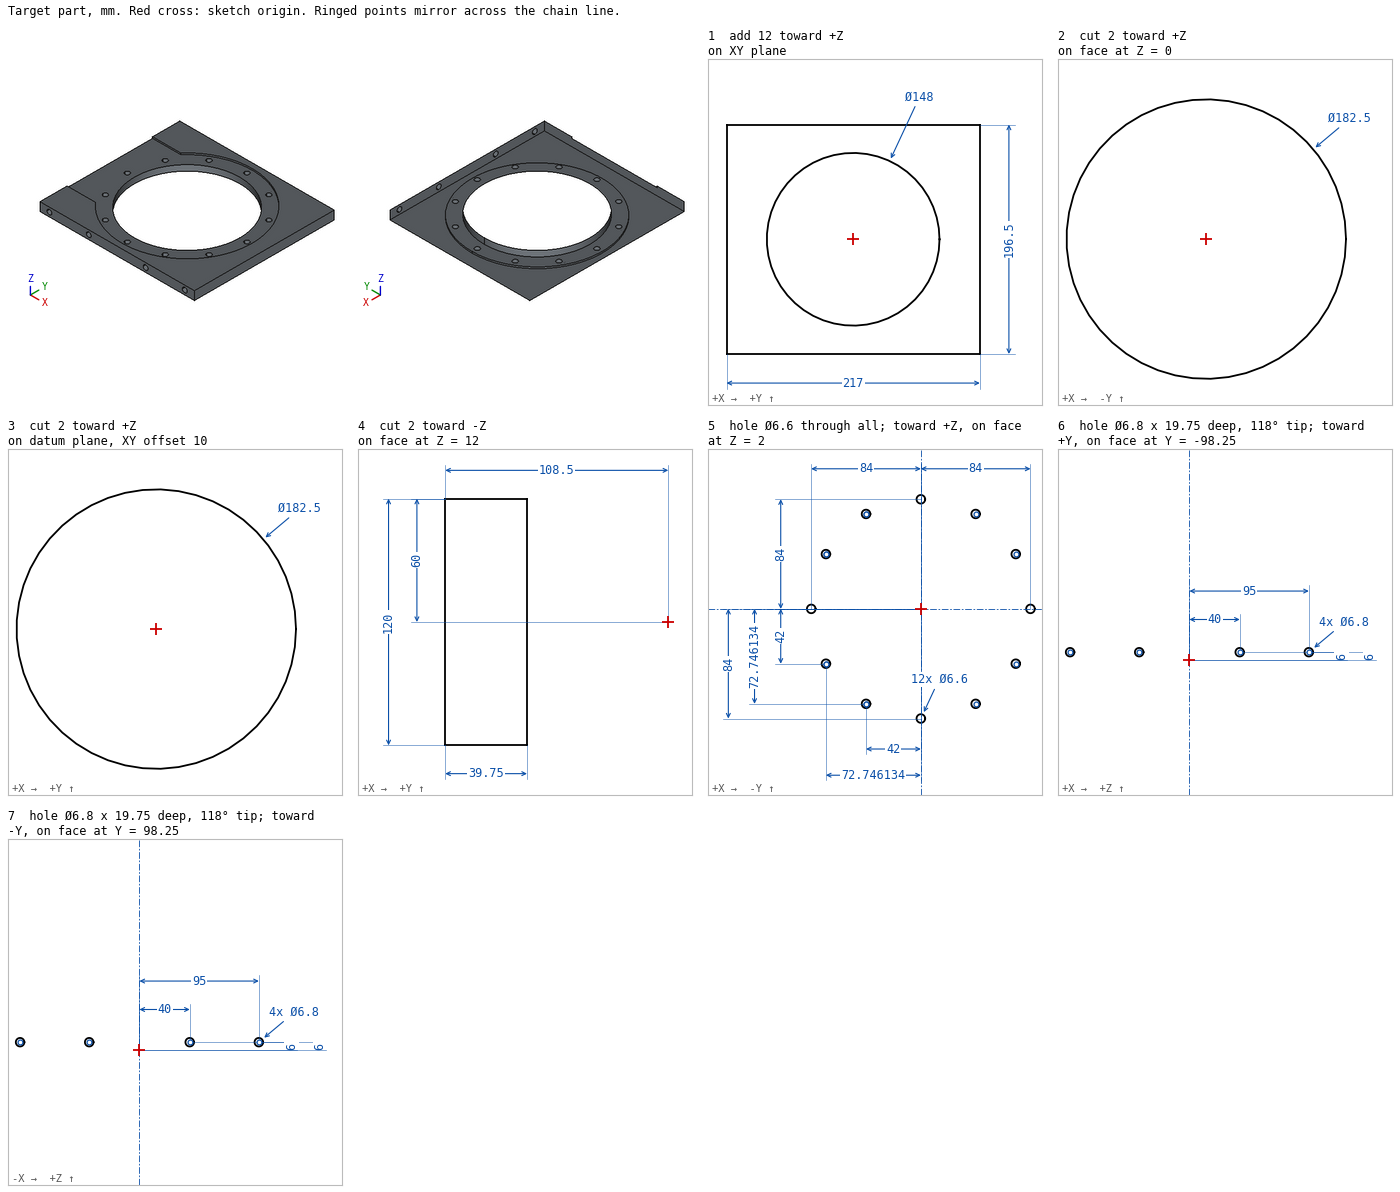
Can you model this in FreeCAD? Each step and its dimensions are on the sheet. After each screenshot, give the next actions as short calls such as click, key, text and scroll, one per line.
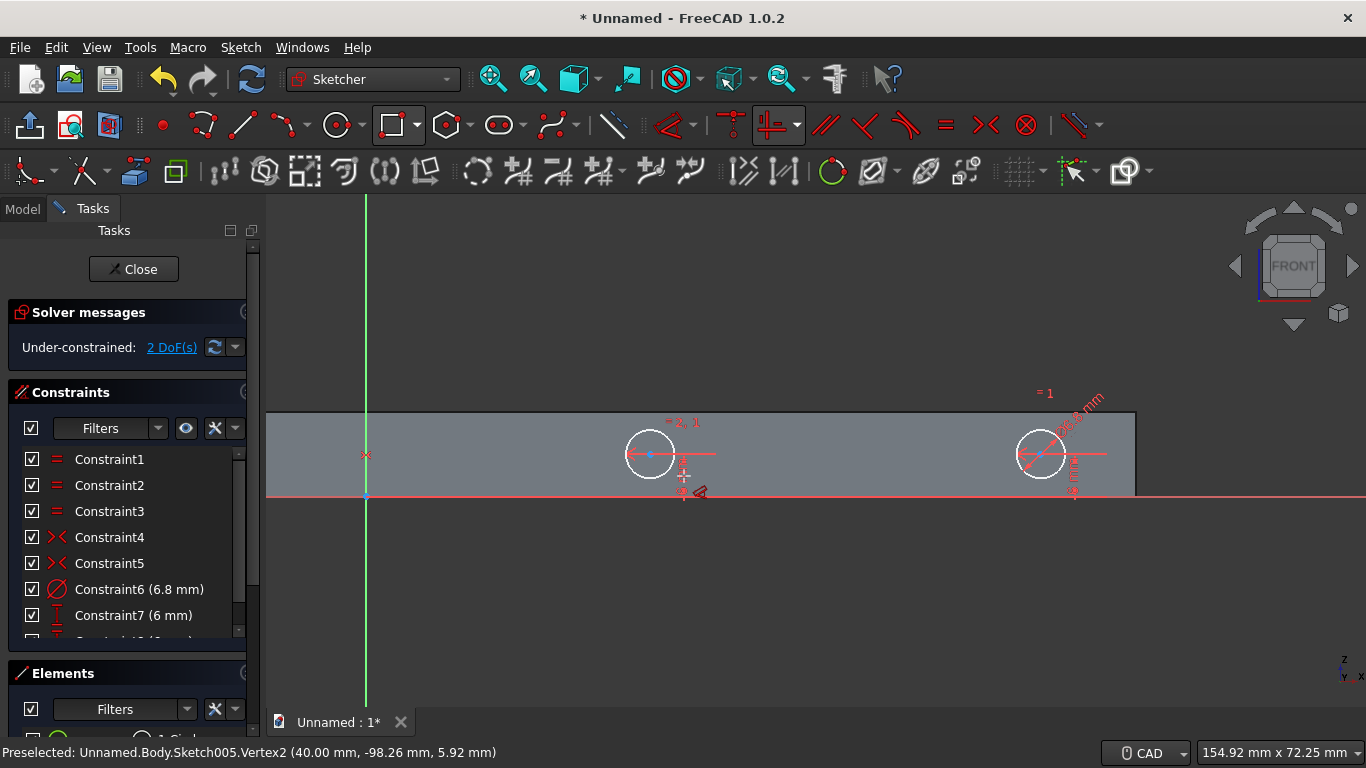
click(1041, 454)
click(703, 531)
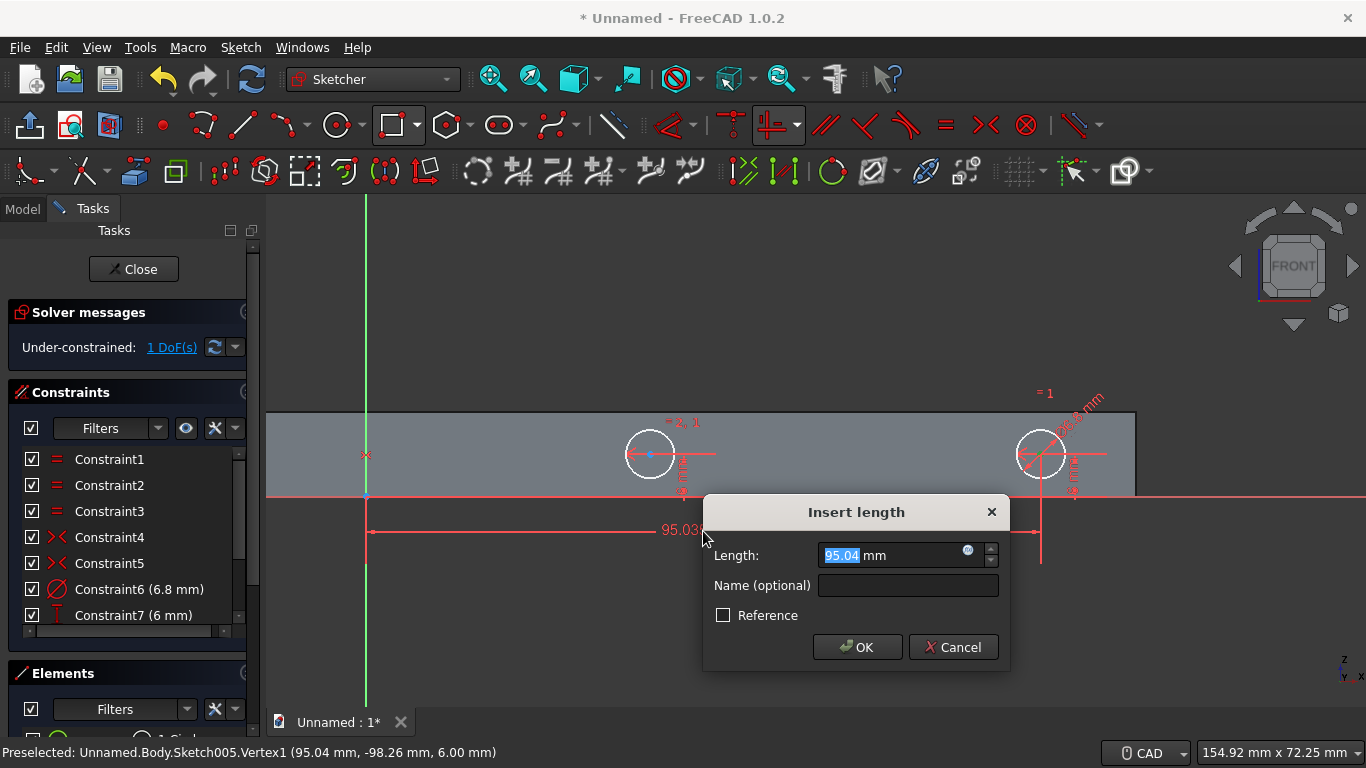
text(95)
key(Return)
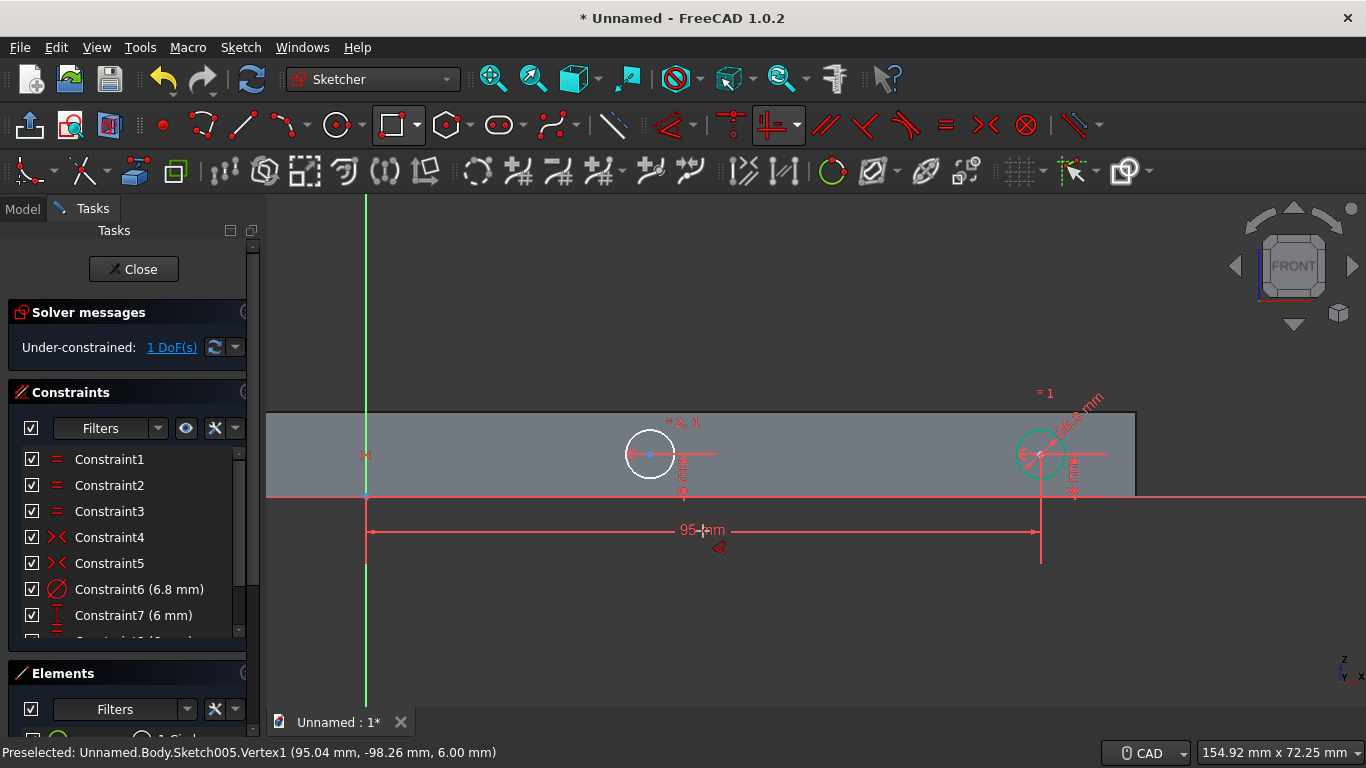
click(650, 454)
click(508, 531)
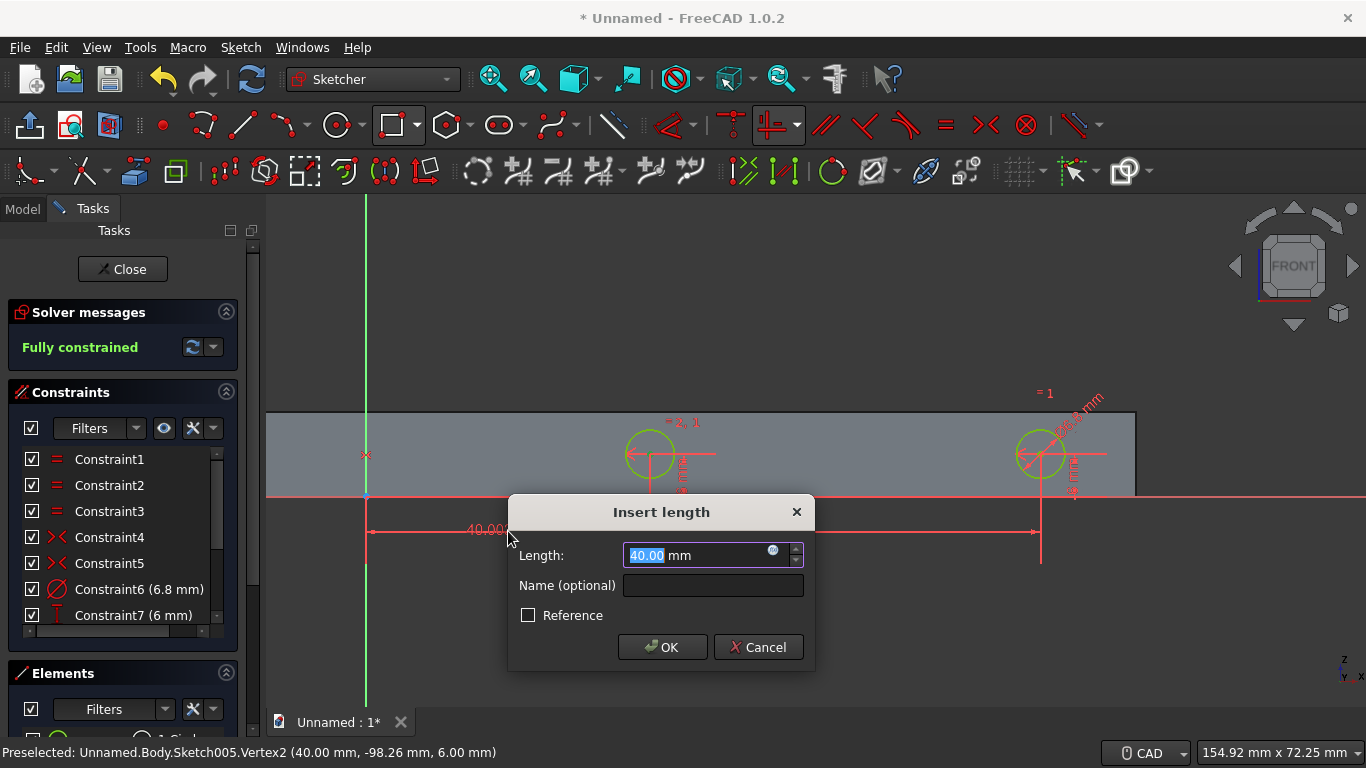
text(40)
key(Return)
key(Escape)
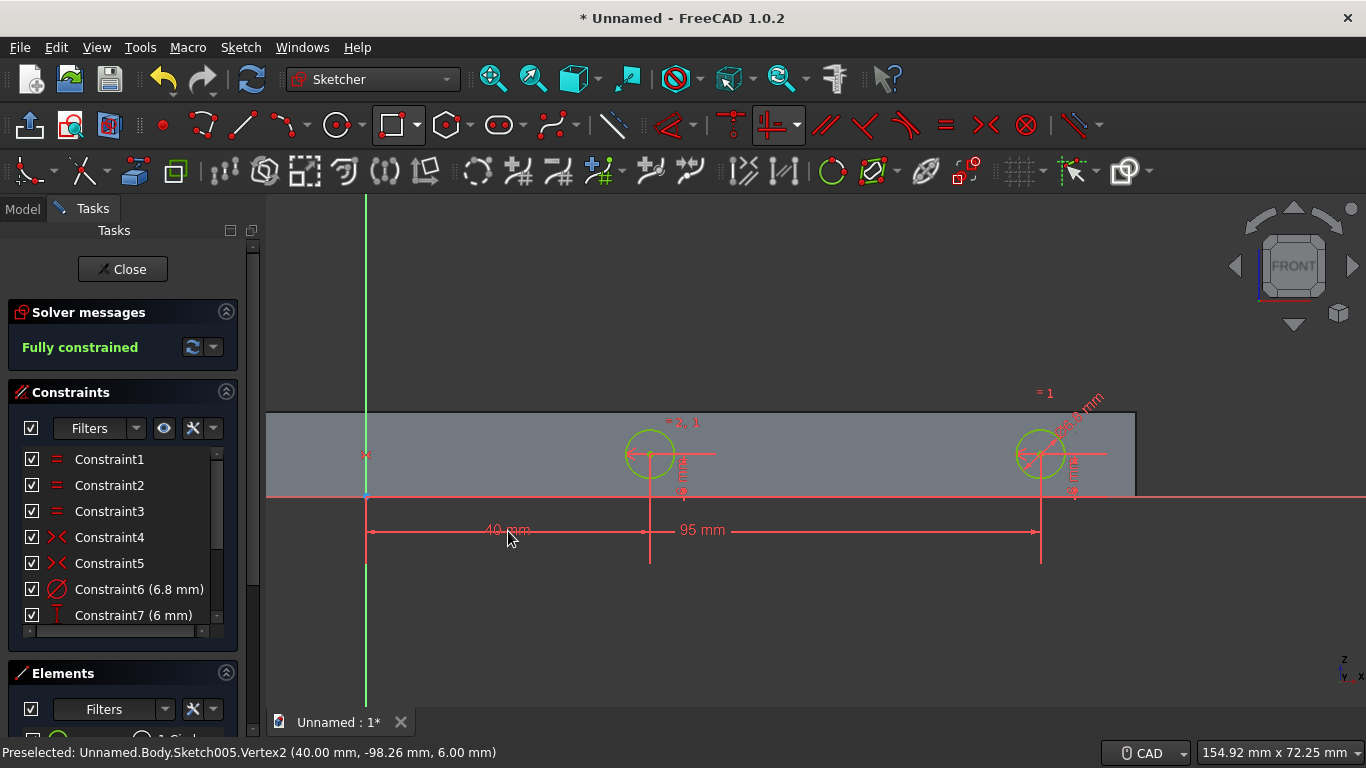
click(123, 269)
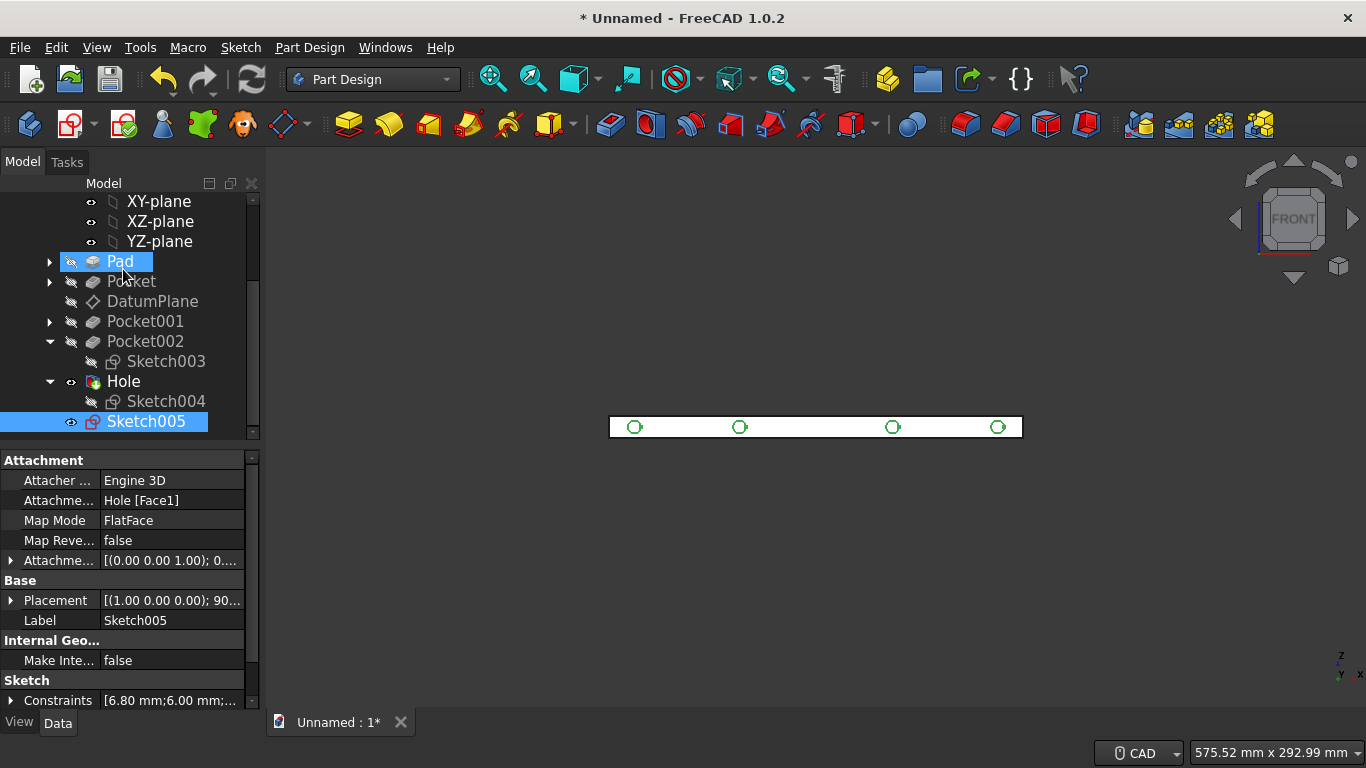
click(652, 124)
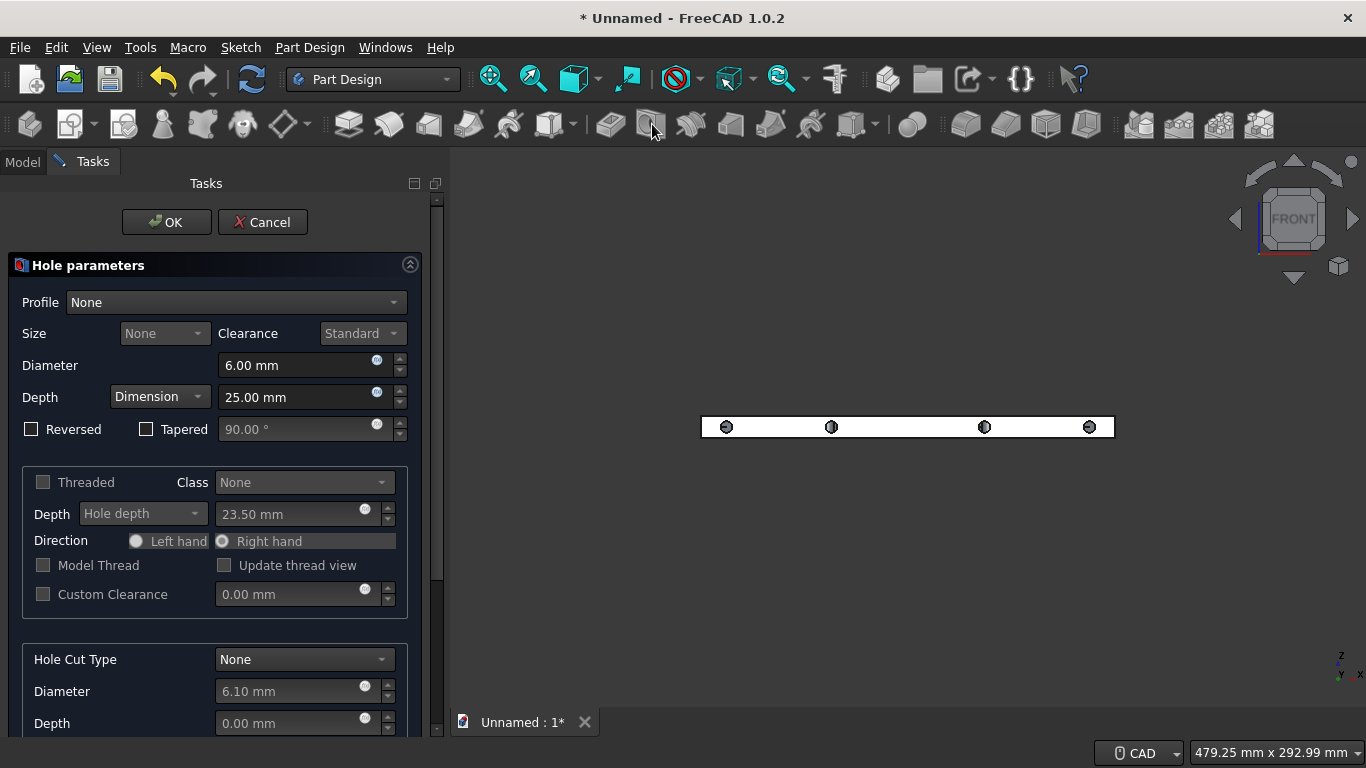
triple_click(305, 365)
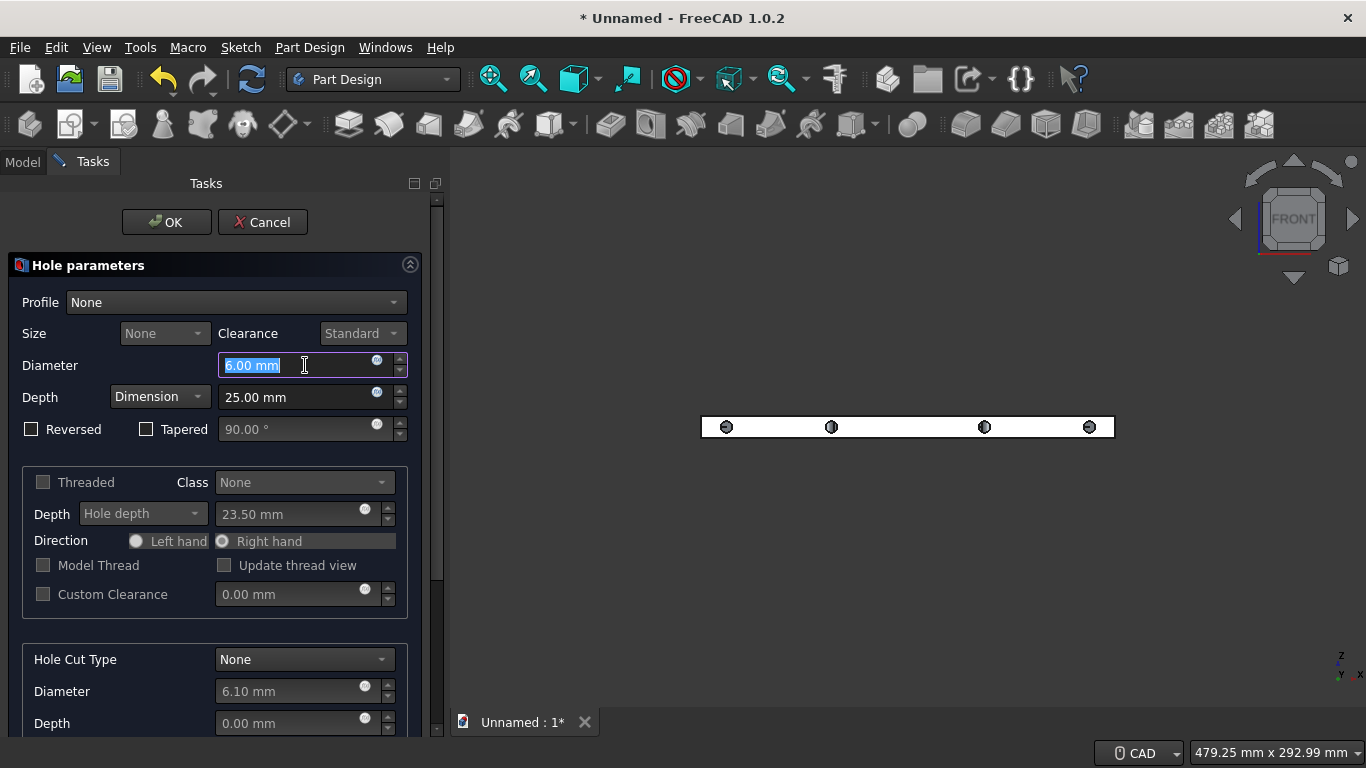
text(6.8)
key(Tab)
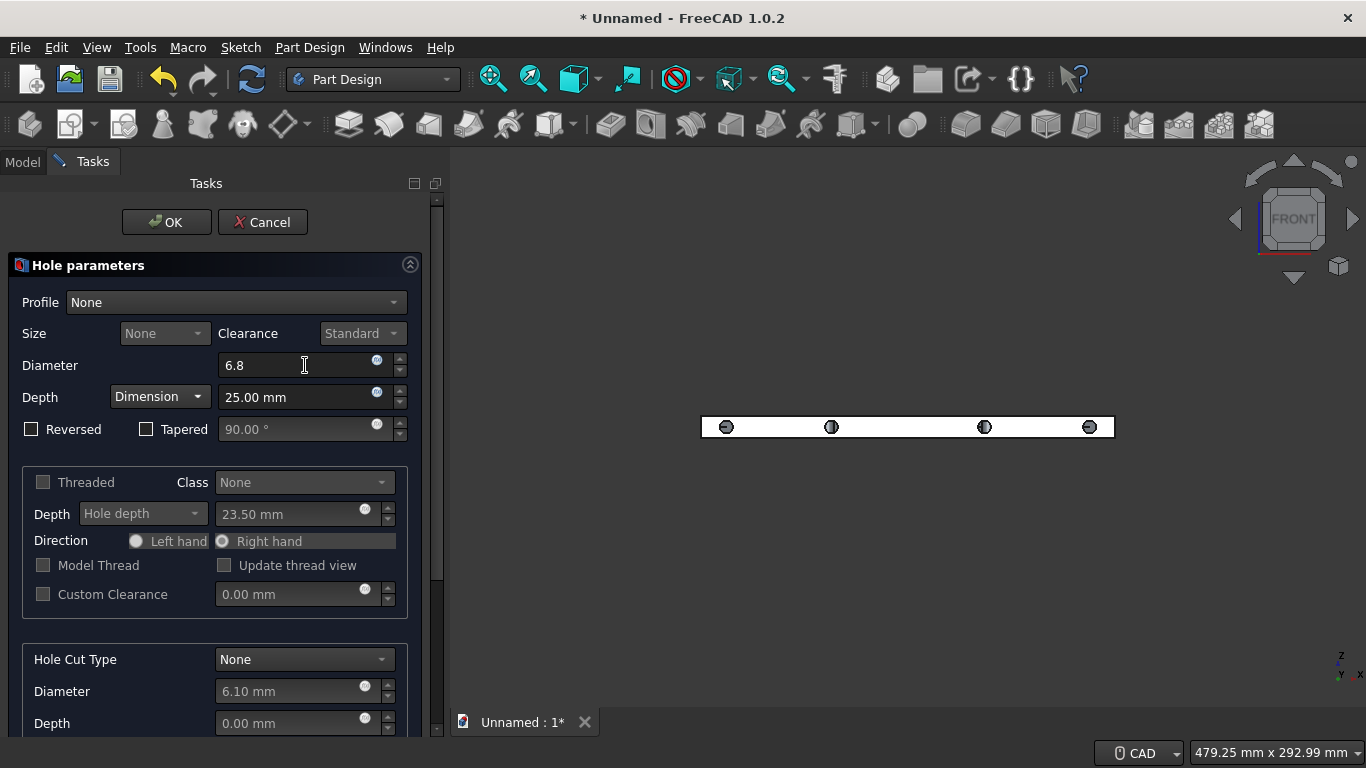
triple_click(305, 397)